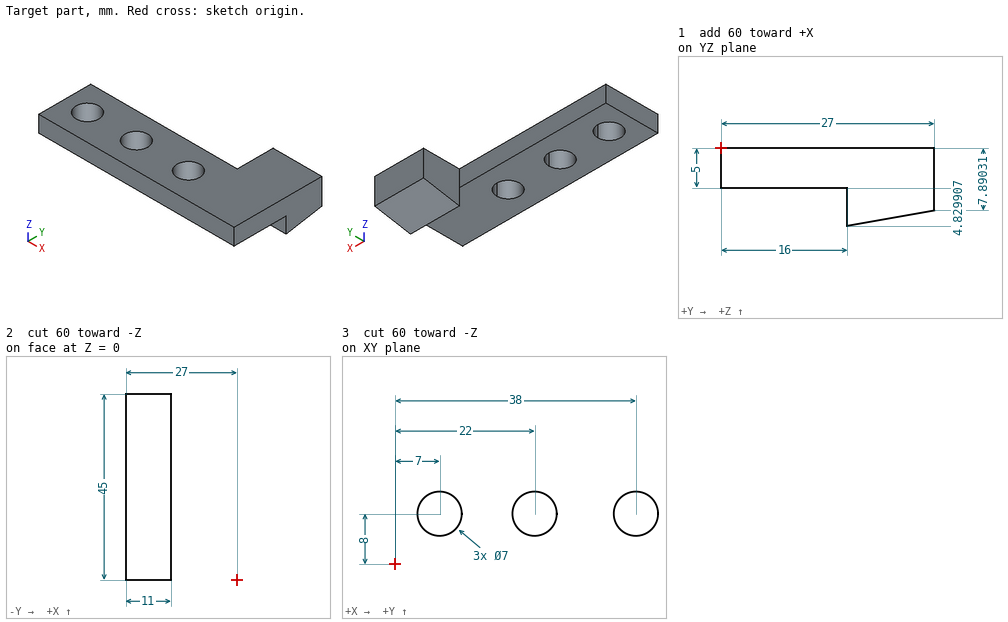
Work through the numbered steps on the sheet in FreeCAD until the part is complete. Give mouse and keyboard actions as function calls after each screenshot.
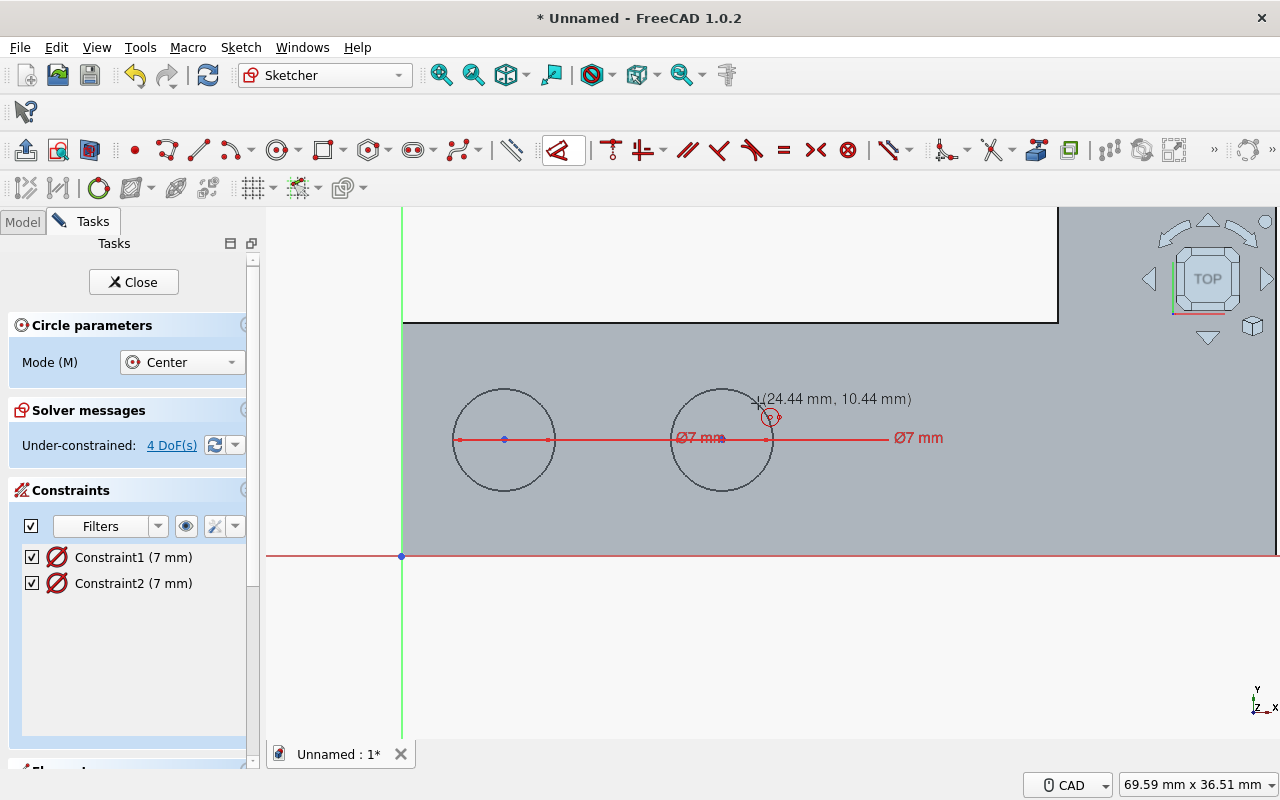
click(956, 439)
move(992, 403)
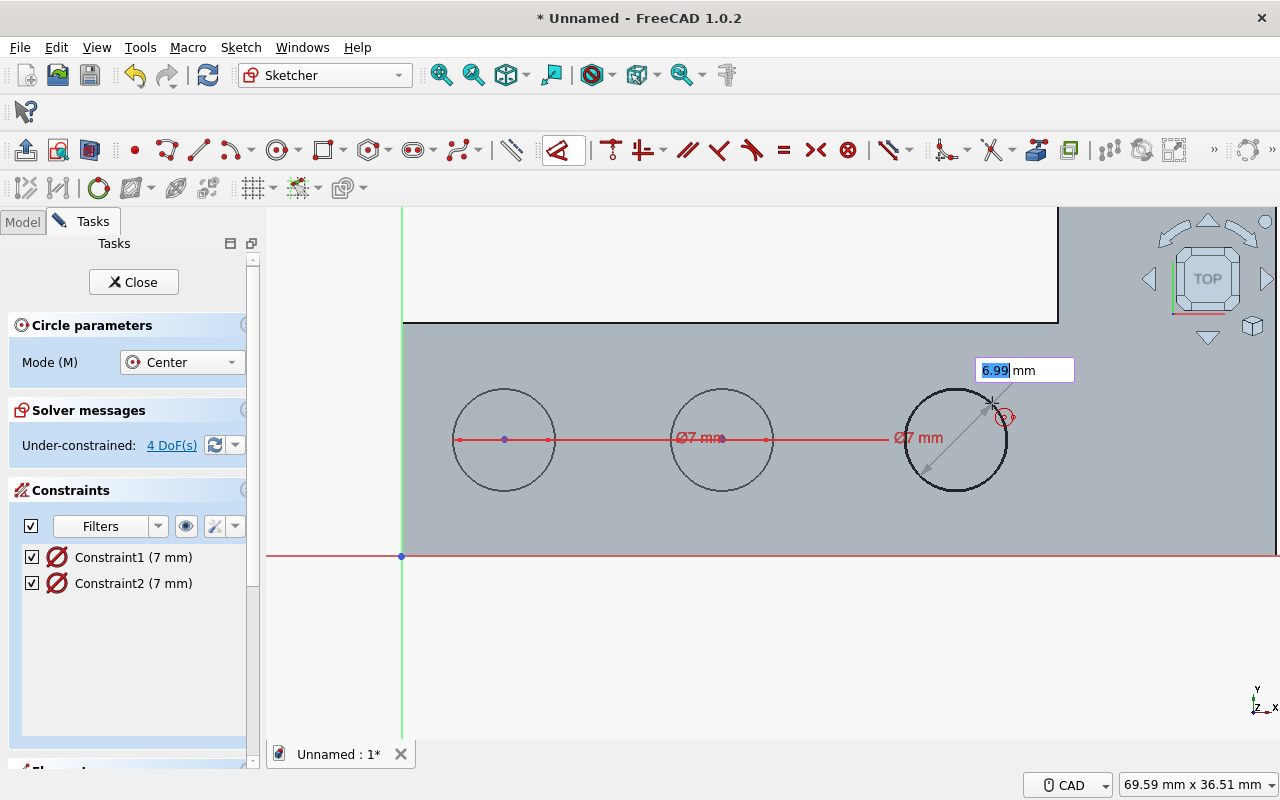
text(7)
key(Return)
key(Escape)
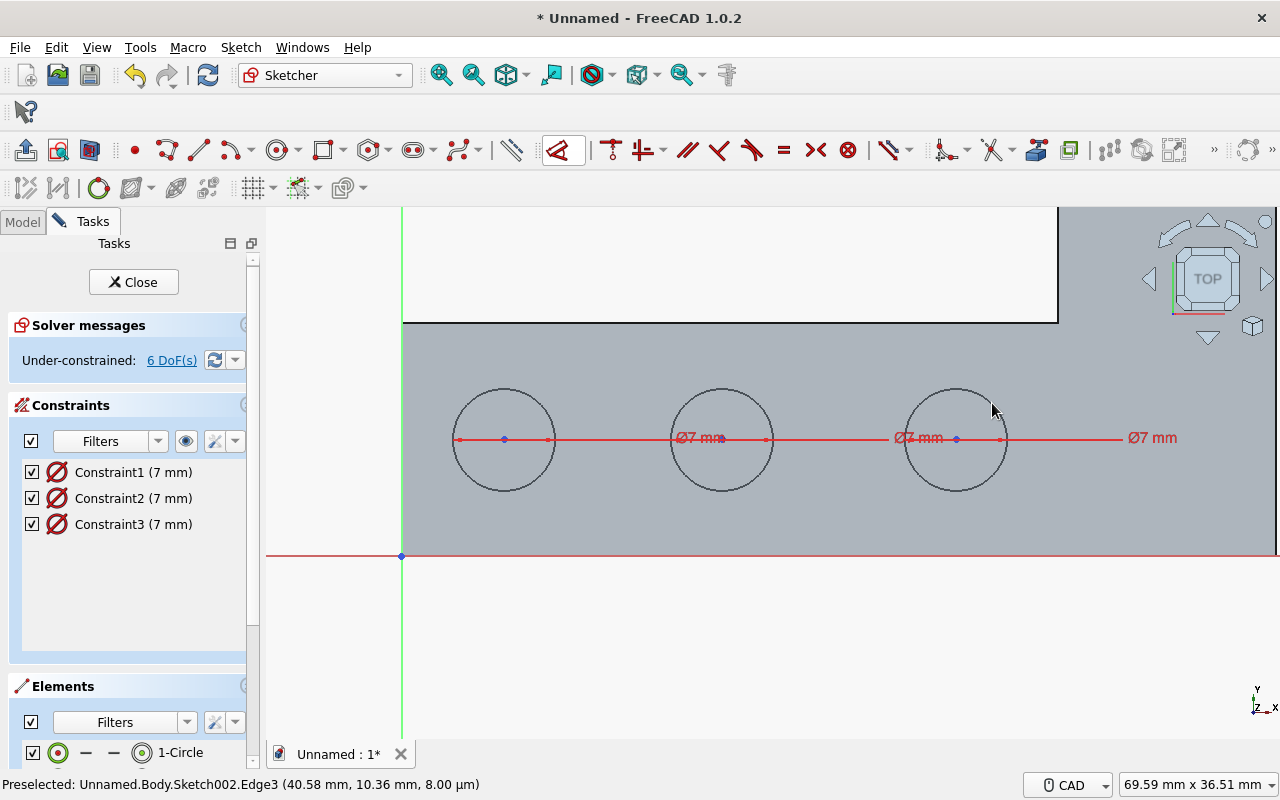
click(504, 440)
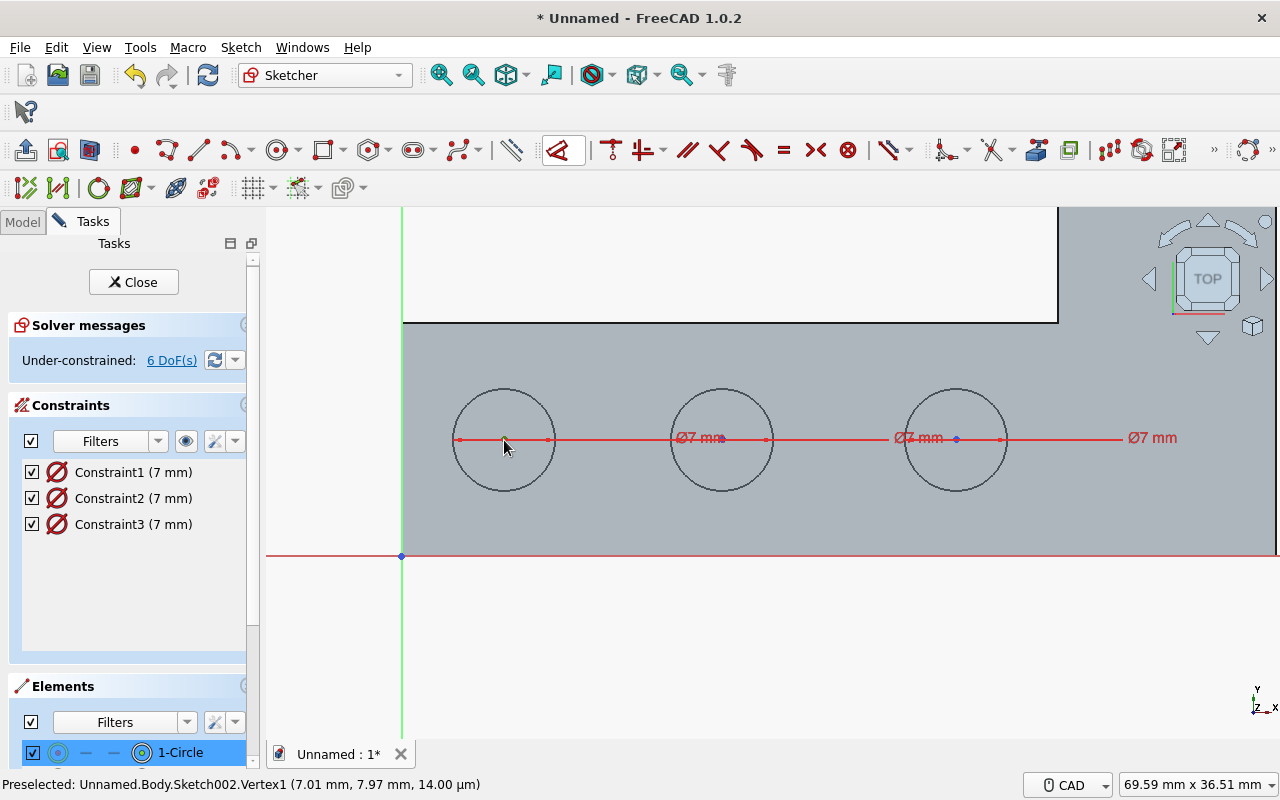
click(722, 440)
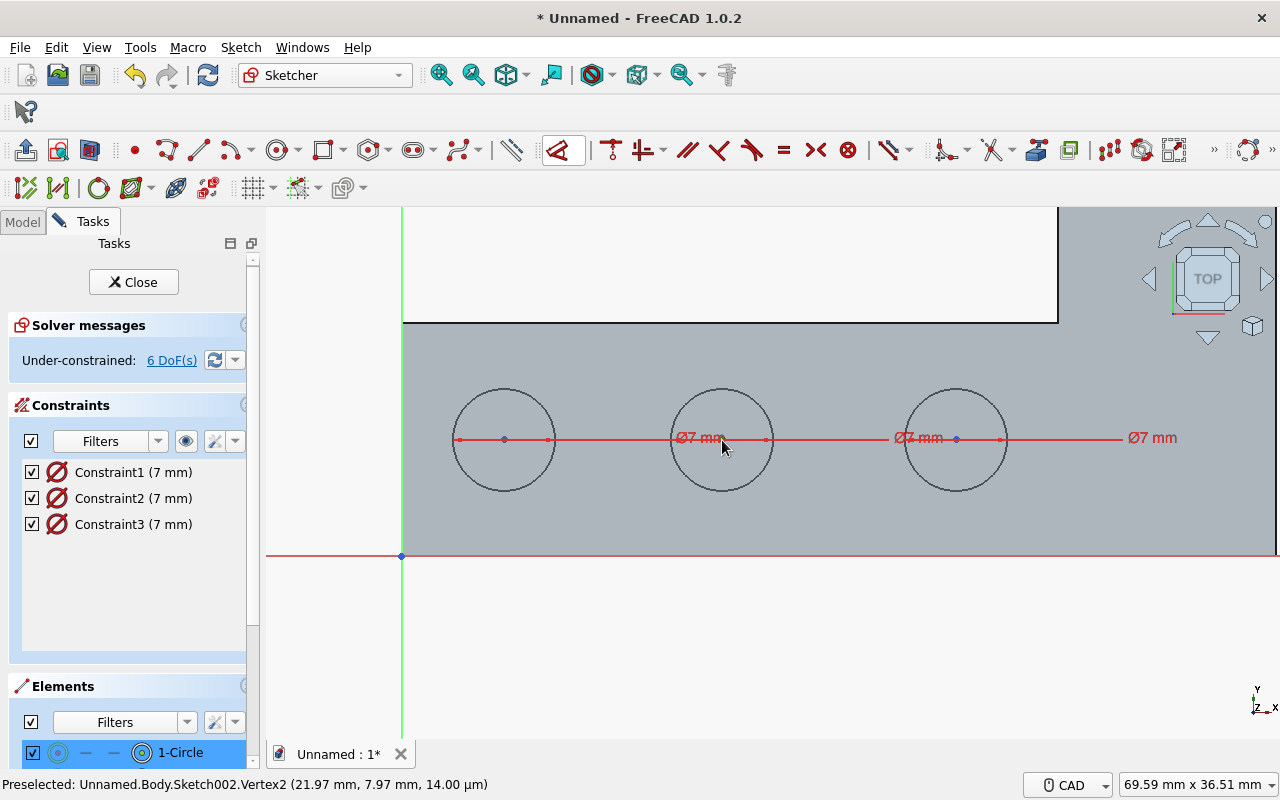
click(666, 150)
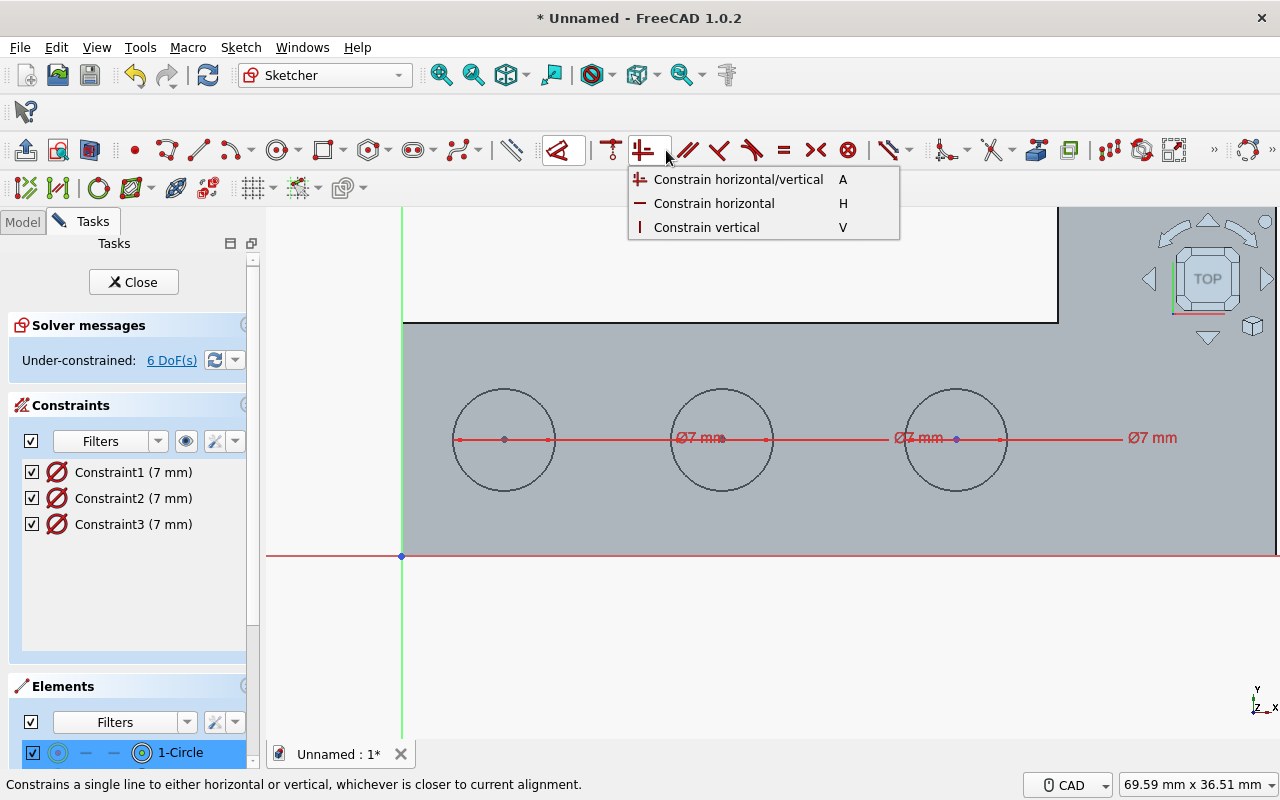
click(764, 203)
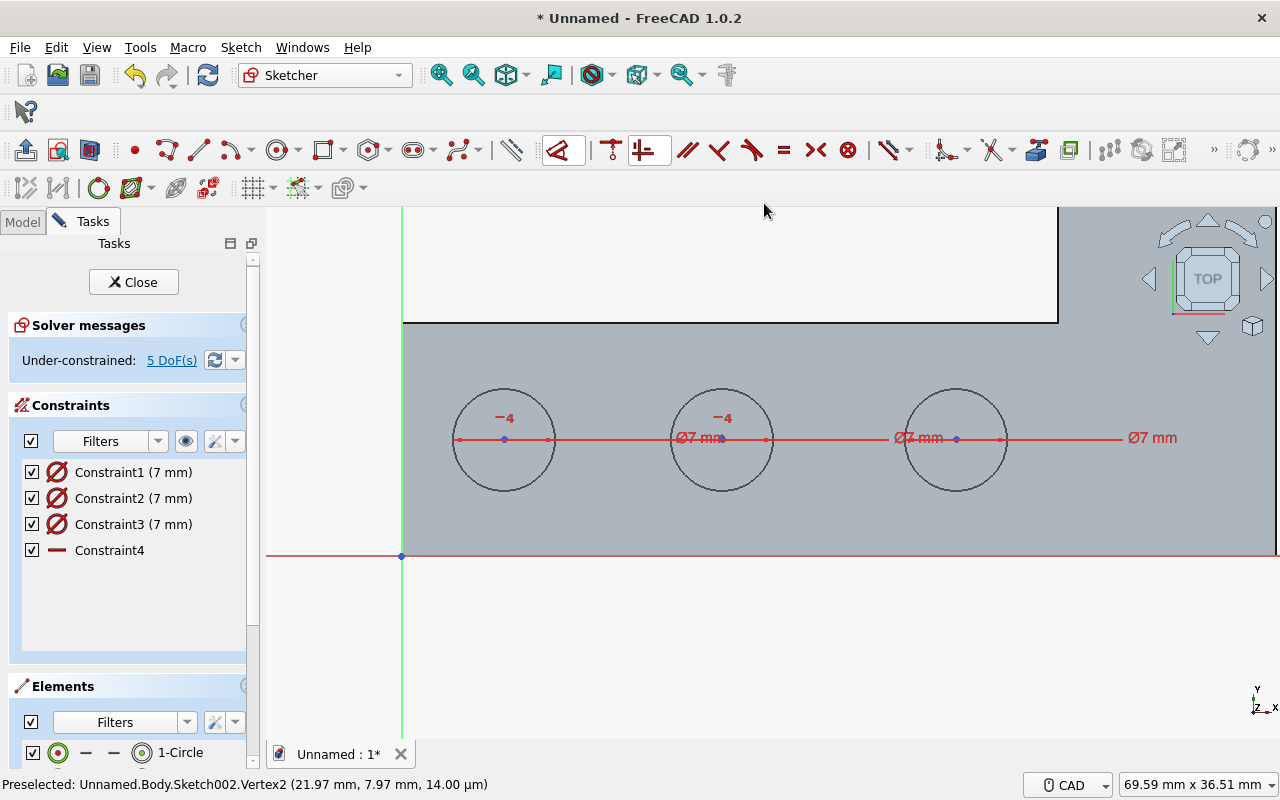
click(722, 440)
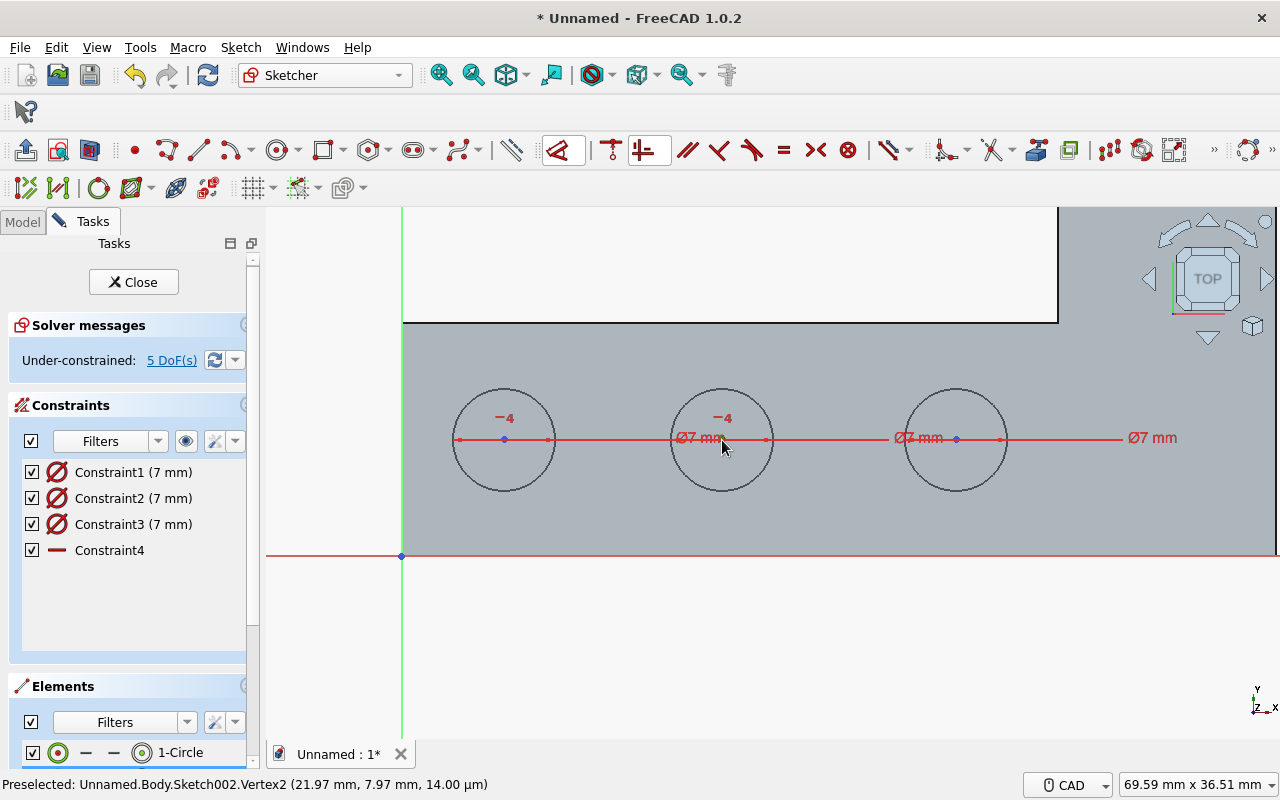
click(956, 440)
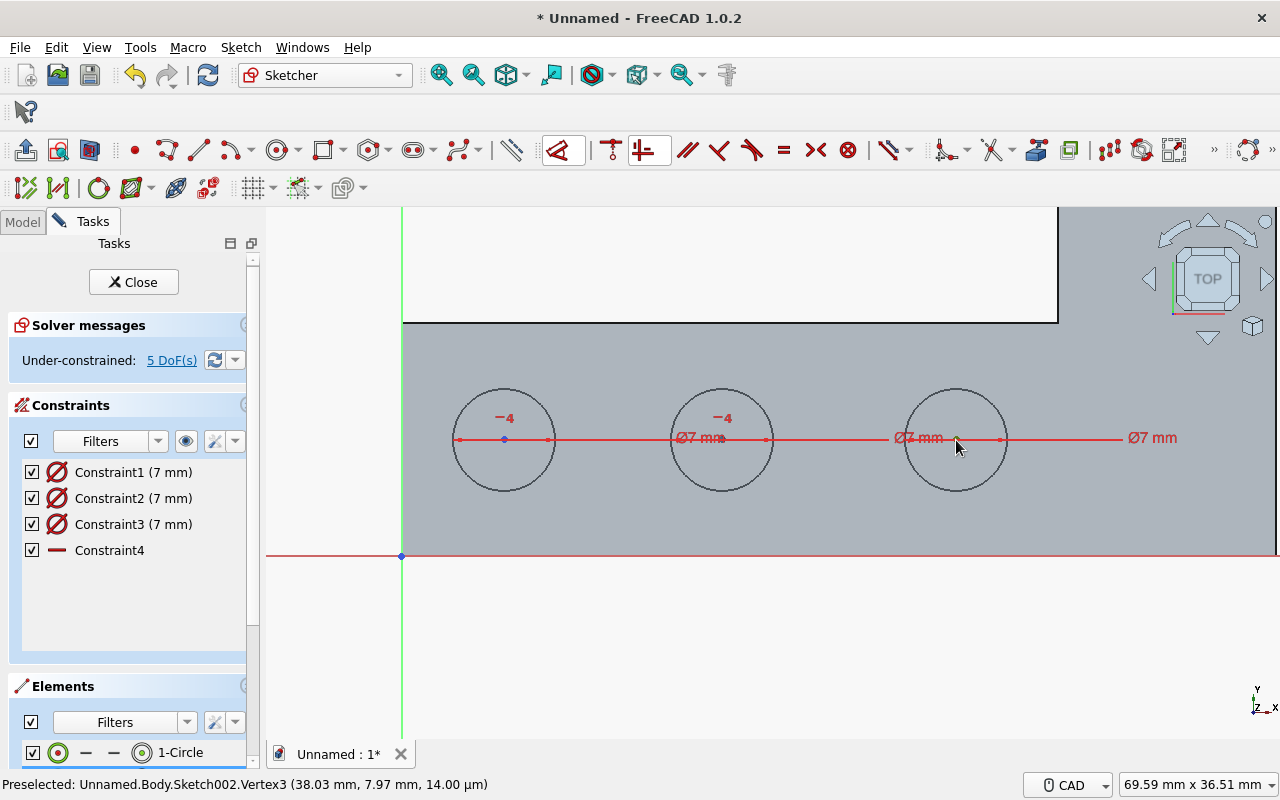
key(h)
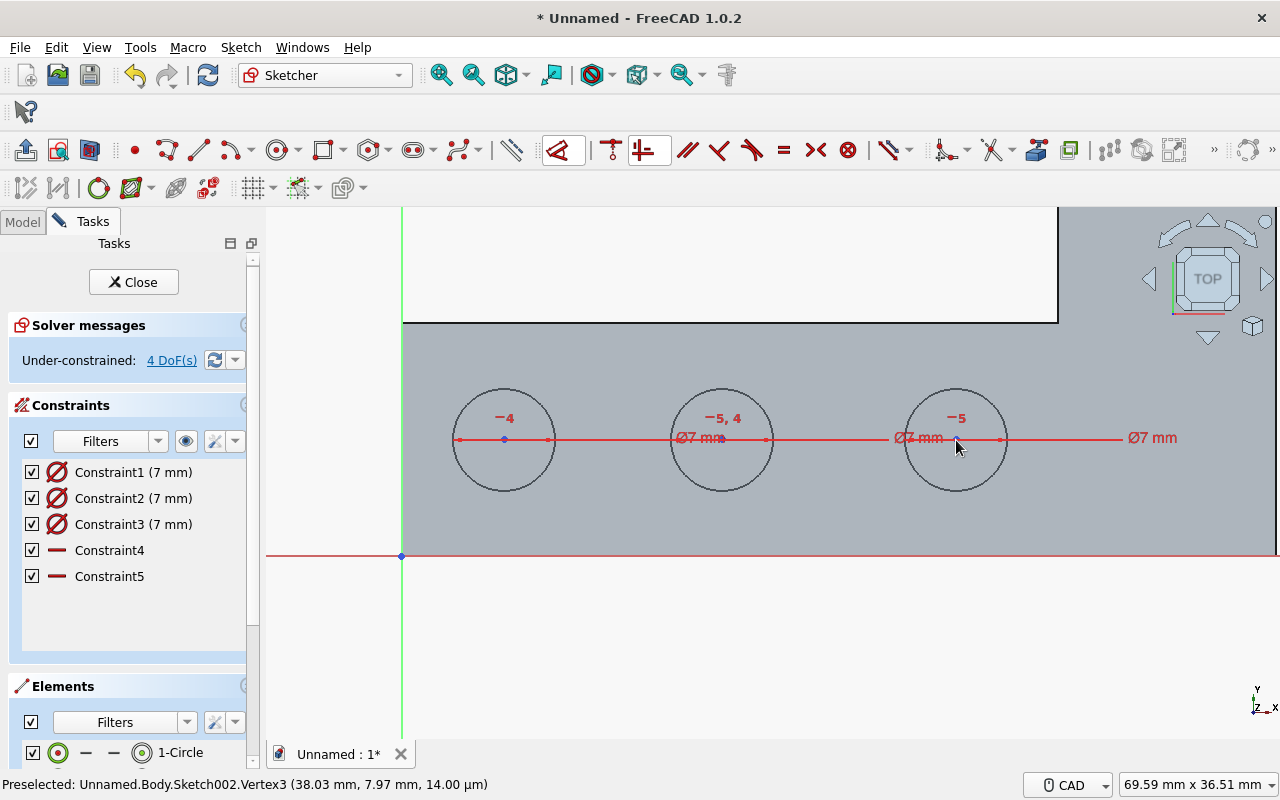
click(504, 440)